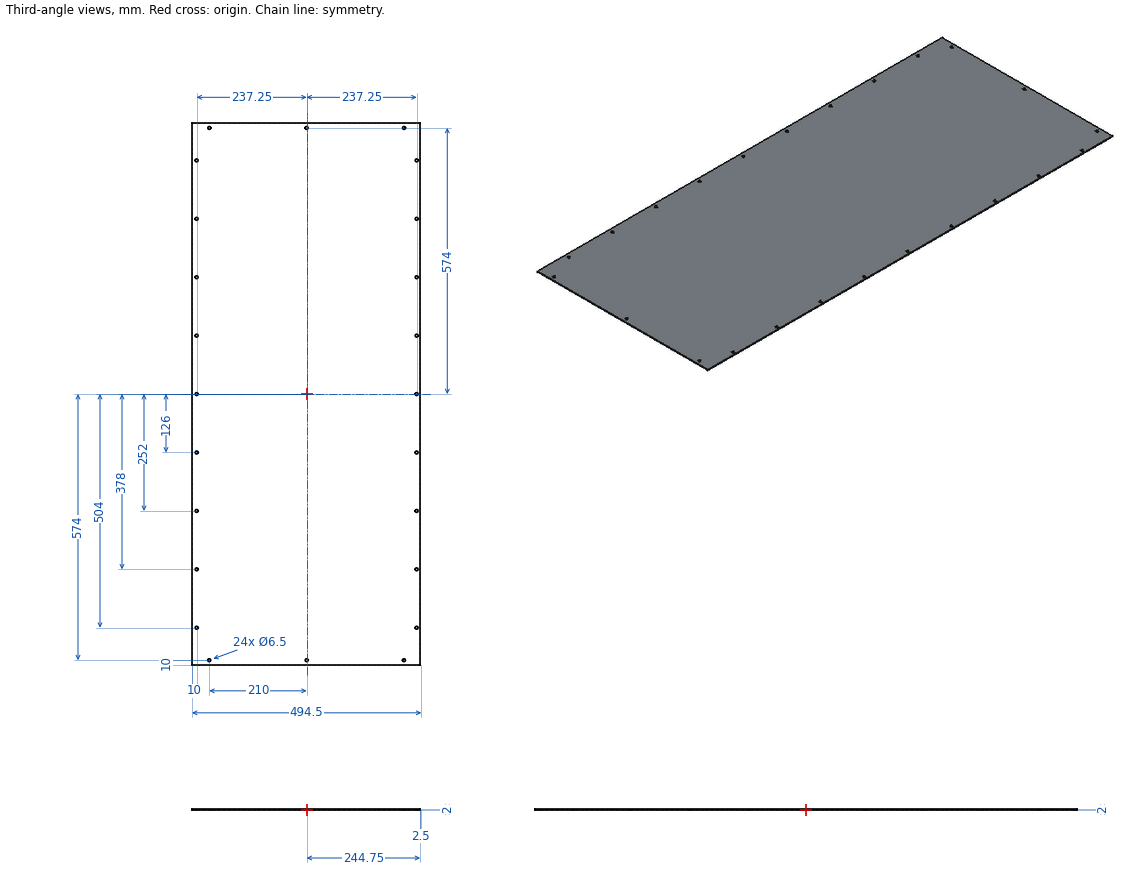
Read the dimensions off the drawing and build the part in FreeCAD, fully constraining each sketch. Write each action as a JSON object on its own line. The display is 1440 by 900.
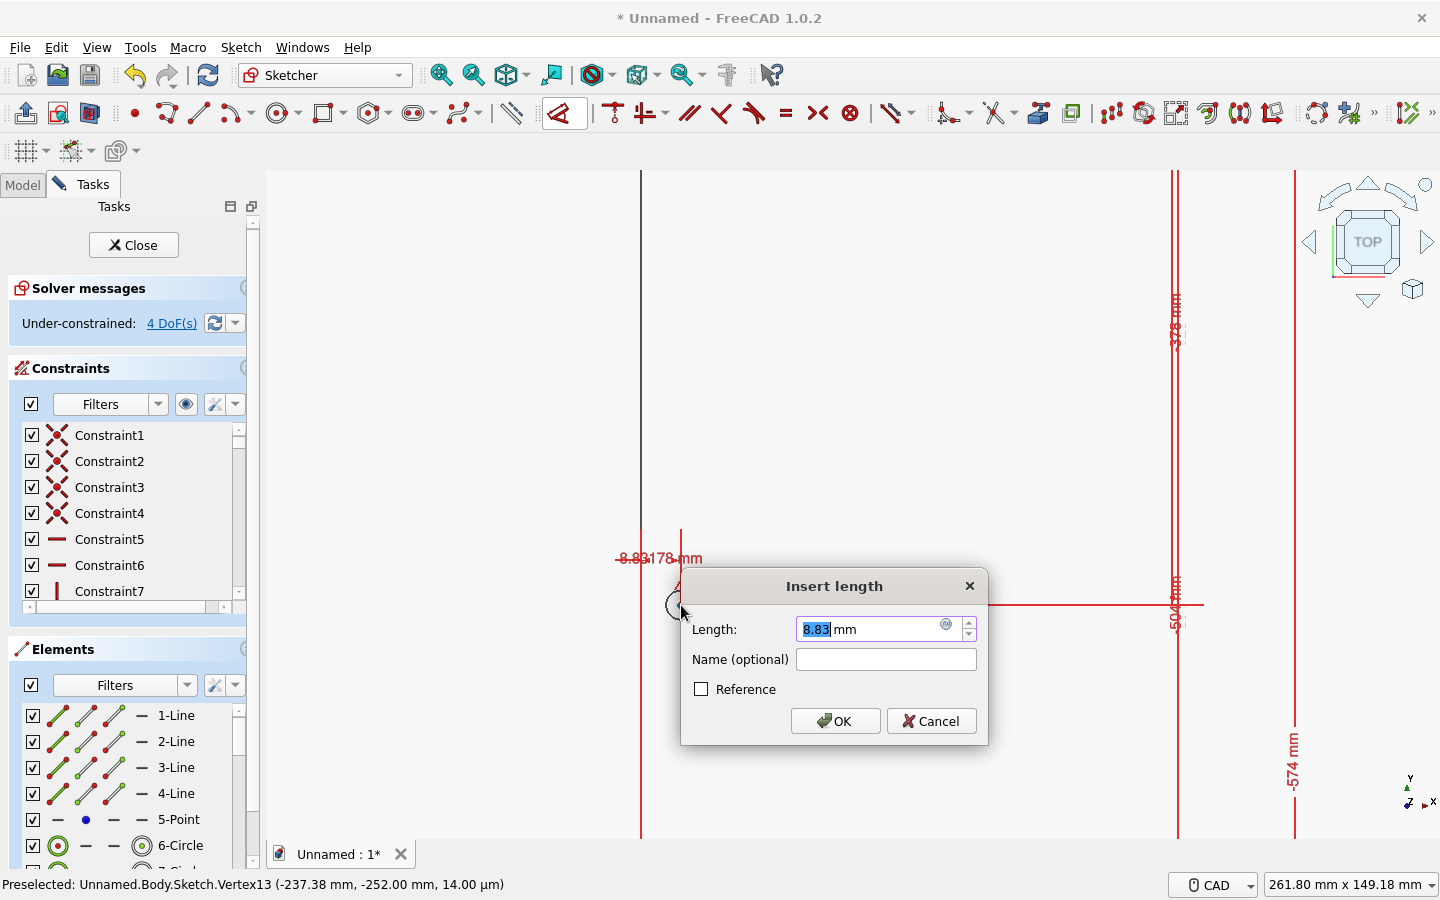
{"action": "type", "text": "10"}
{"action": "key", "text": "Return"}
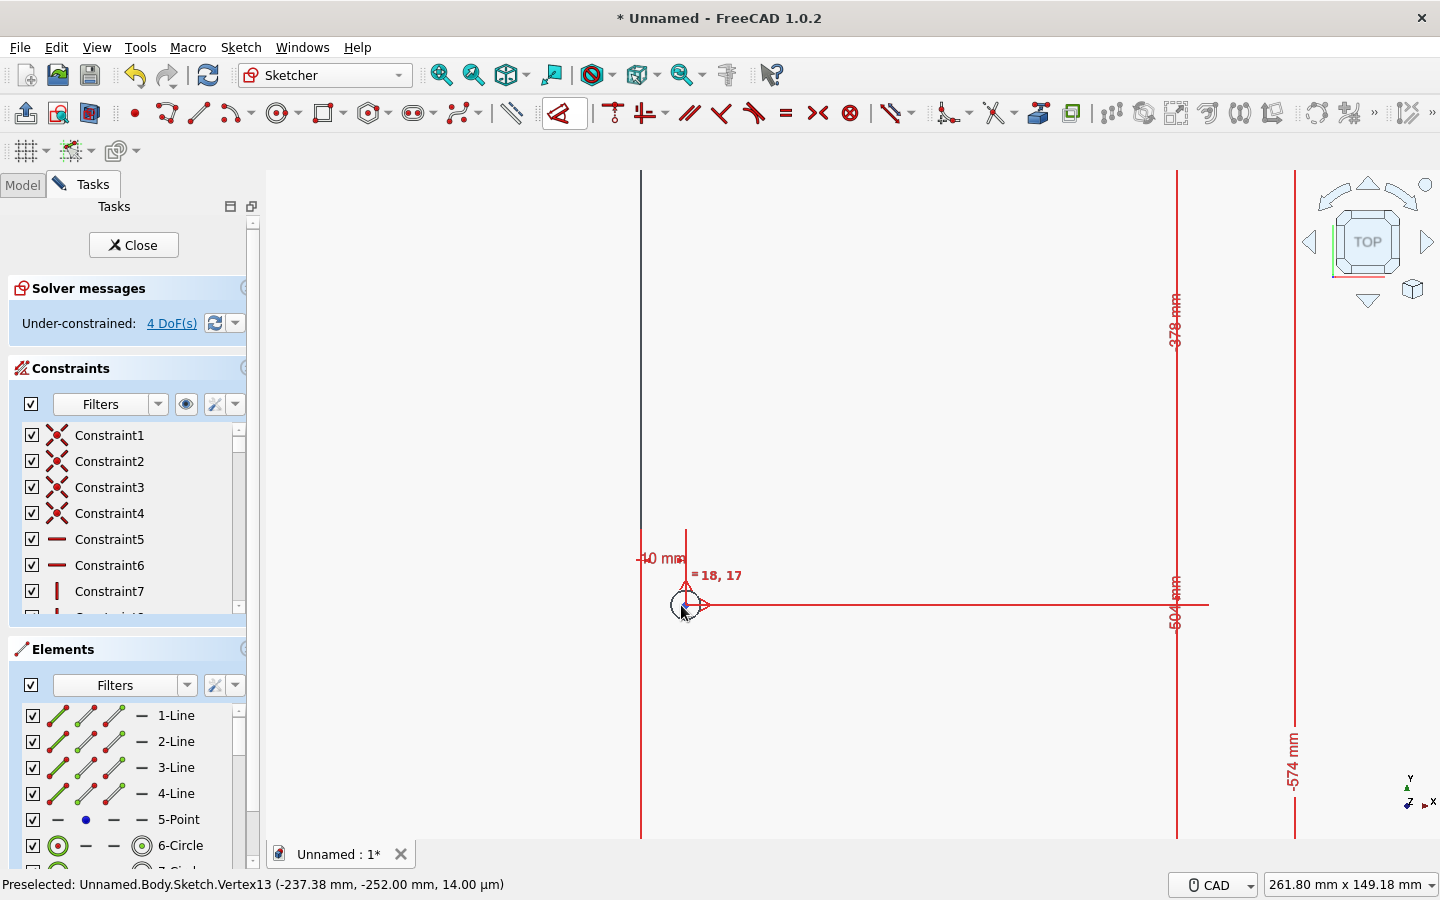
{"action": "scroll", "coordinate": [689, 607], "scroll_direction": "down", "scroll_amount": 12}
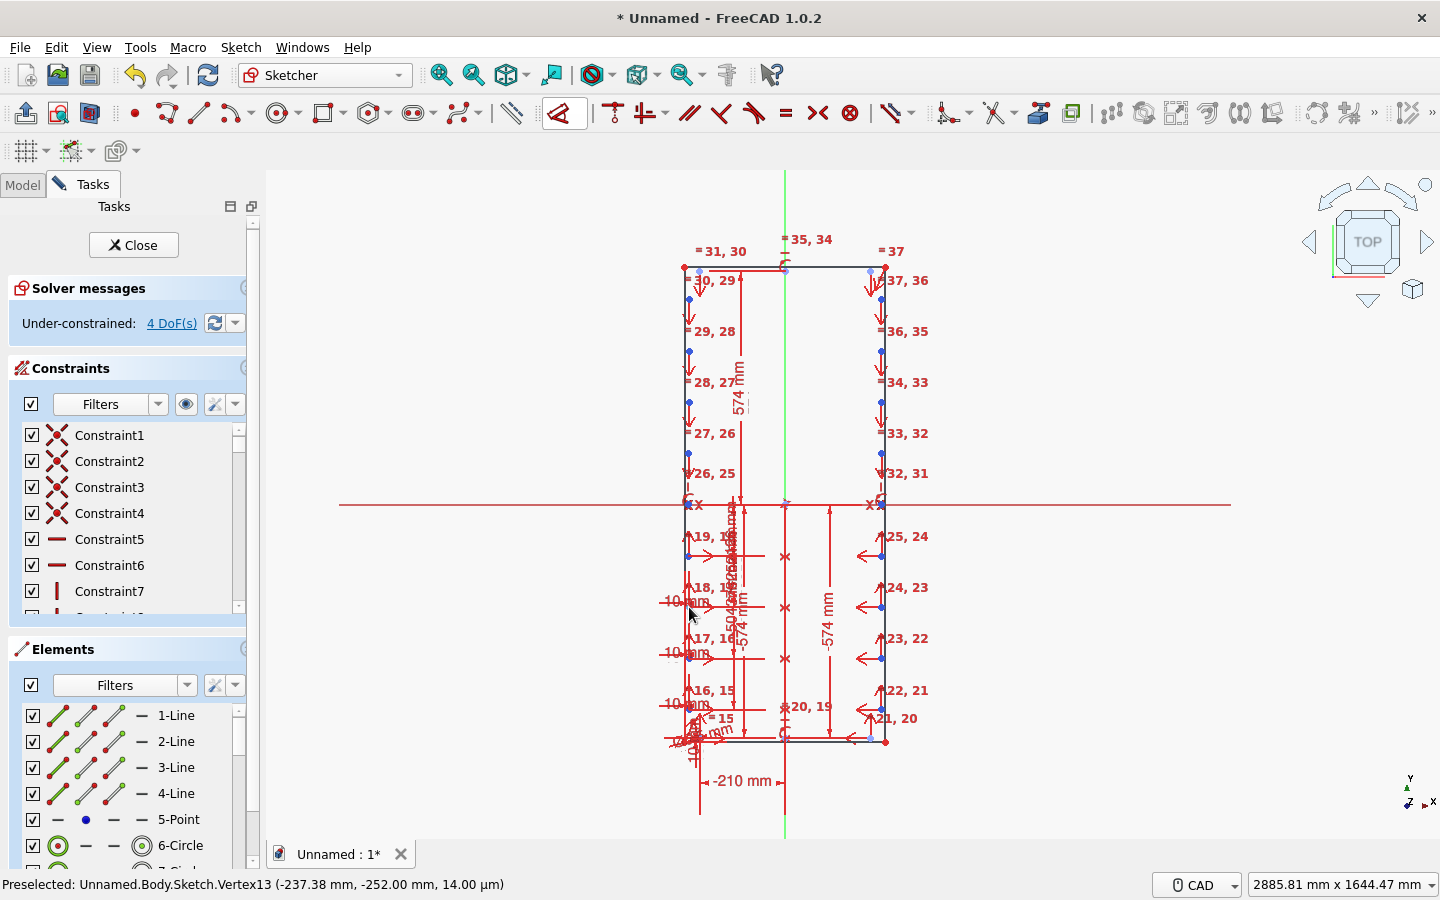
{"action": "scroll", "coordinate": [685, 742], "scroll_direction": "up", "scroll_amount": 12}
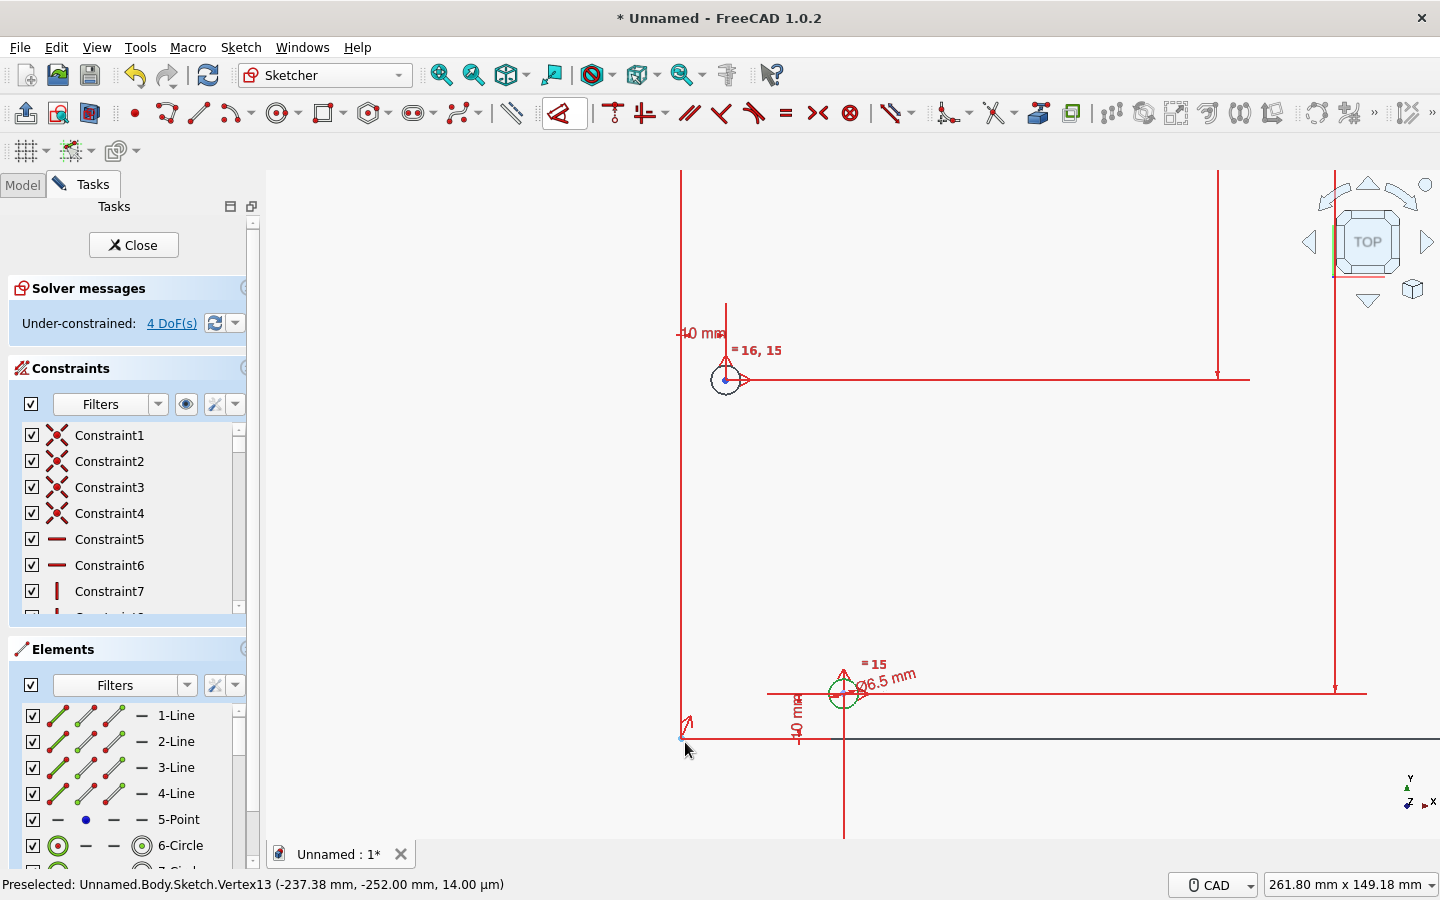
{"action": "left_click", "coordinate": [681, 739]}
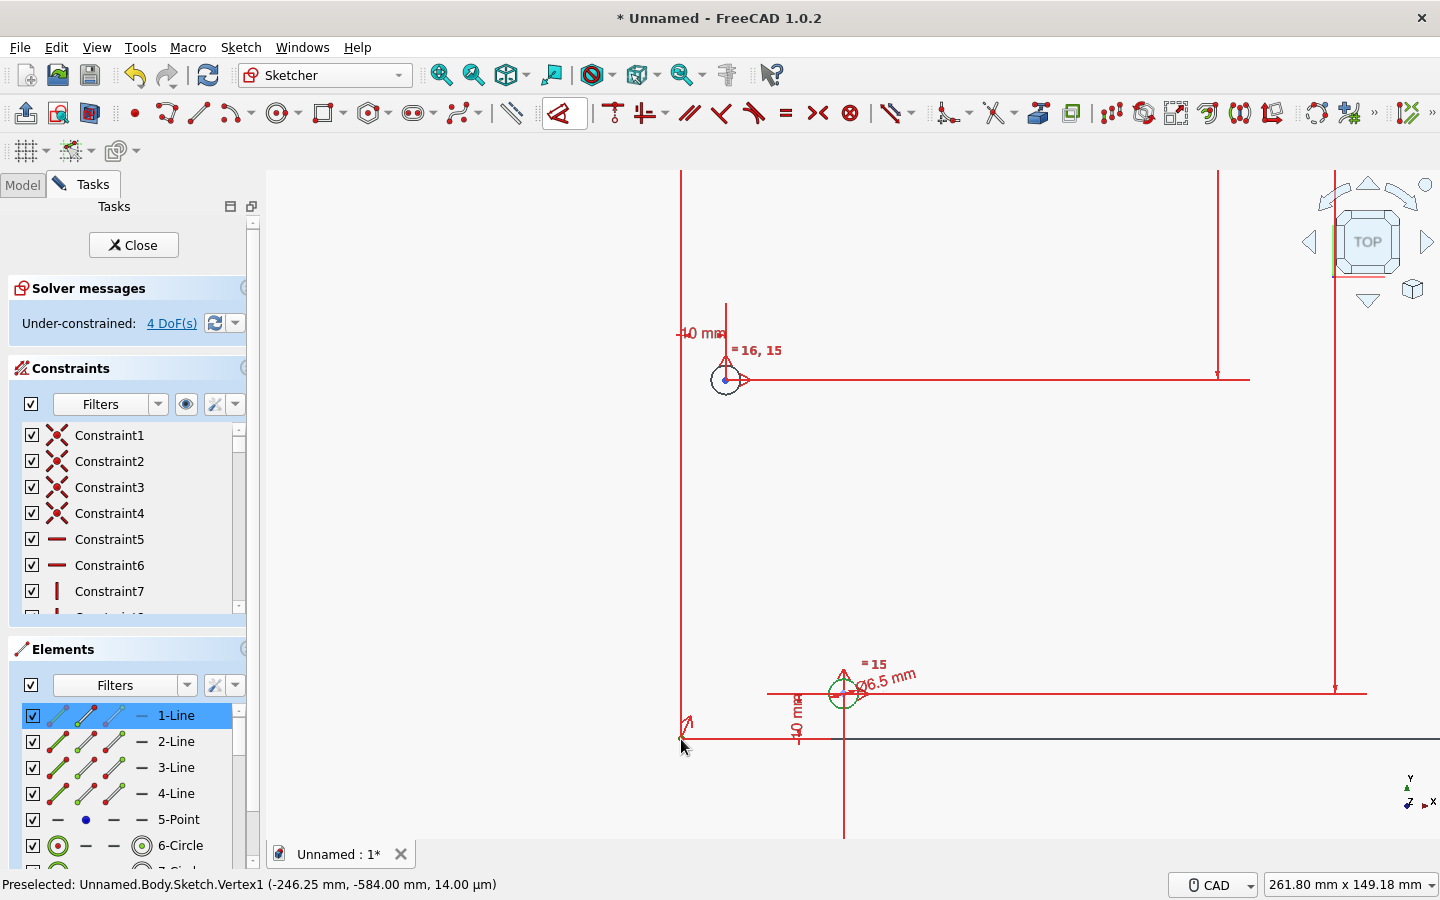
{"action": "scroll", "coordinate": [685, 742], "scroll_direction": "down", "scroll_amount": 12}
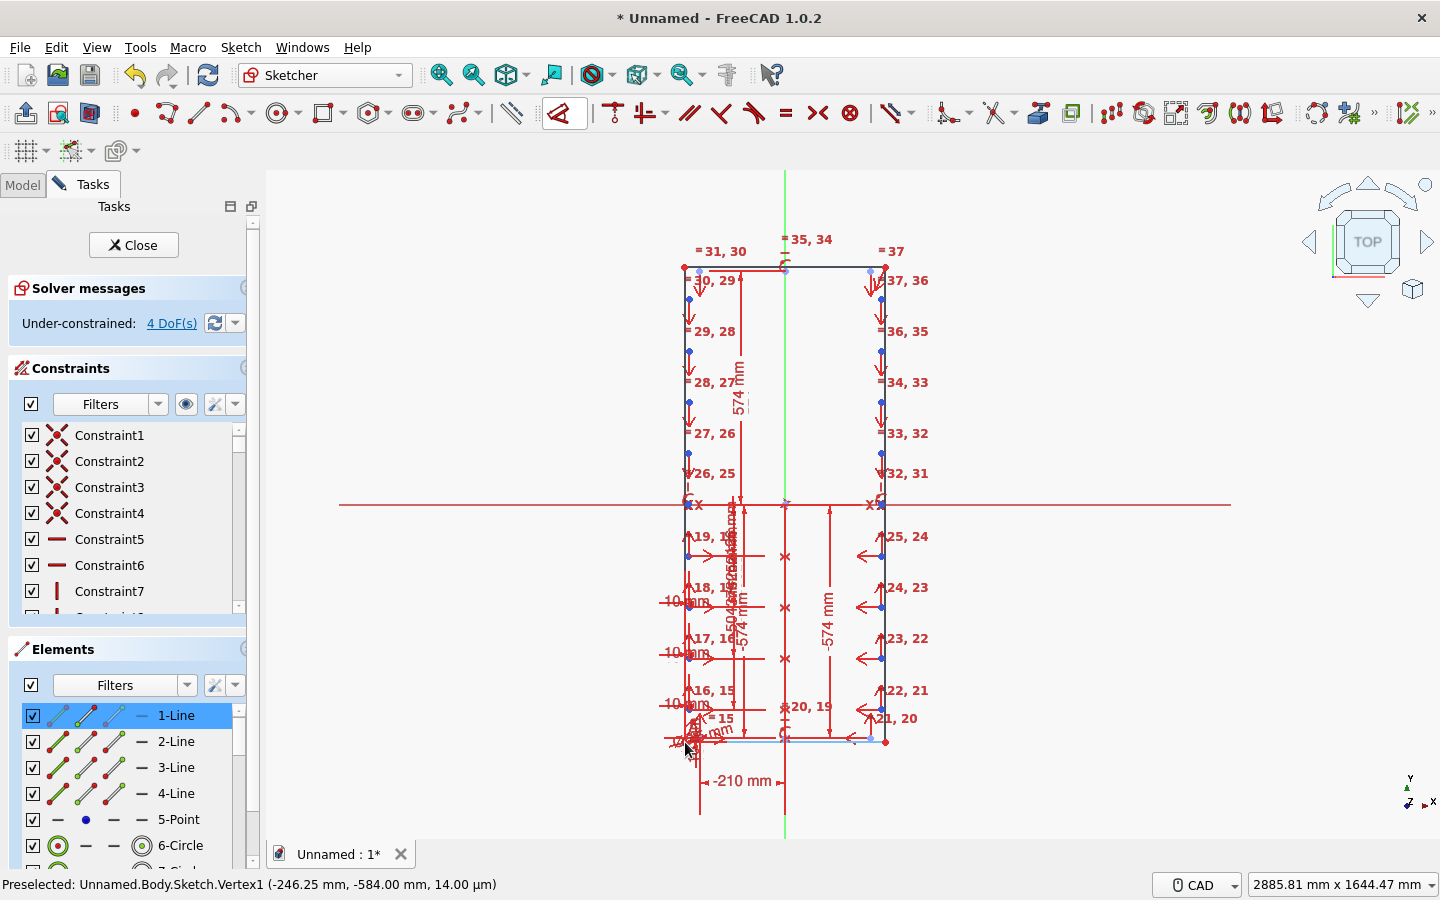
{"action": "scroll", "coordinate": [689, 556], "scroll_direction": "up", "scroll_amount": 12}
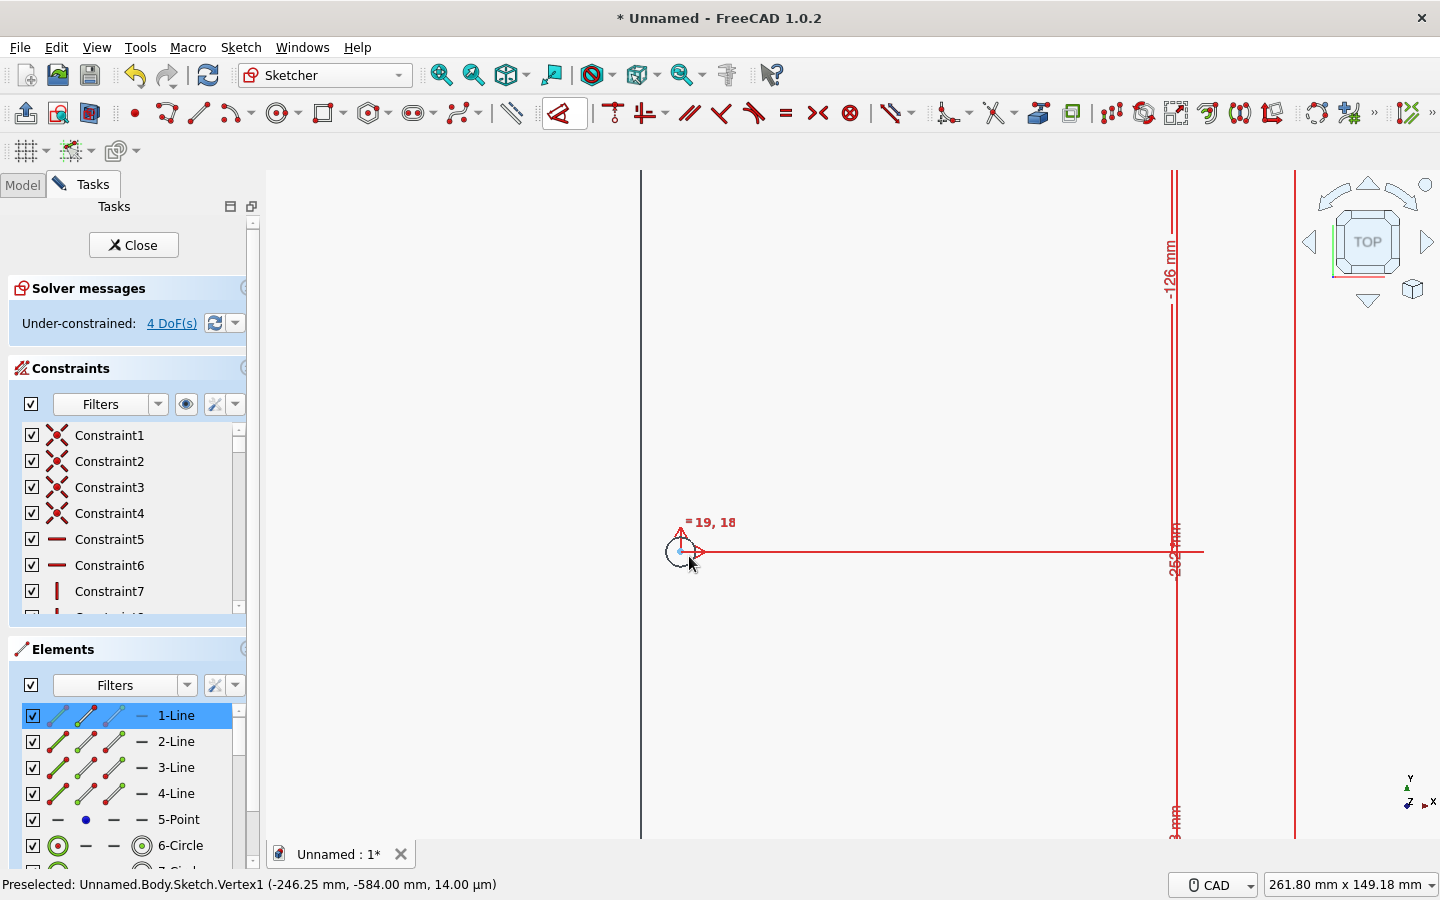
{"action": "left_click", "coordinate": [681, 552]}